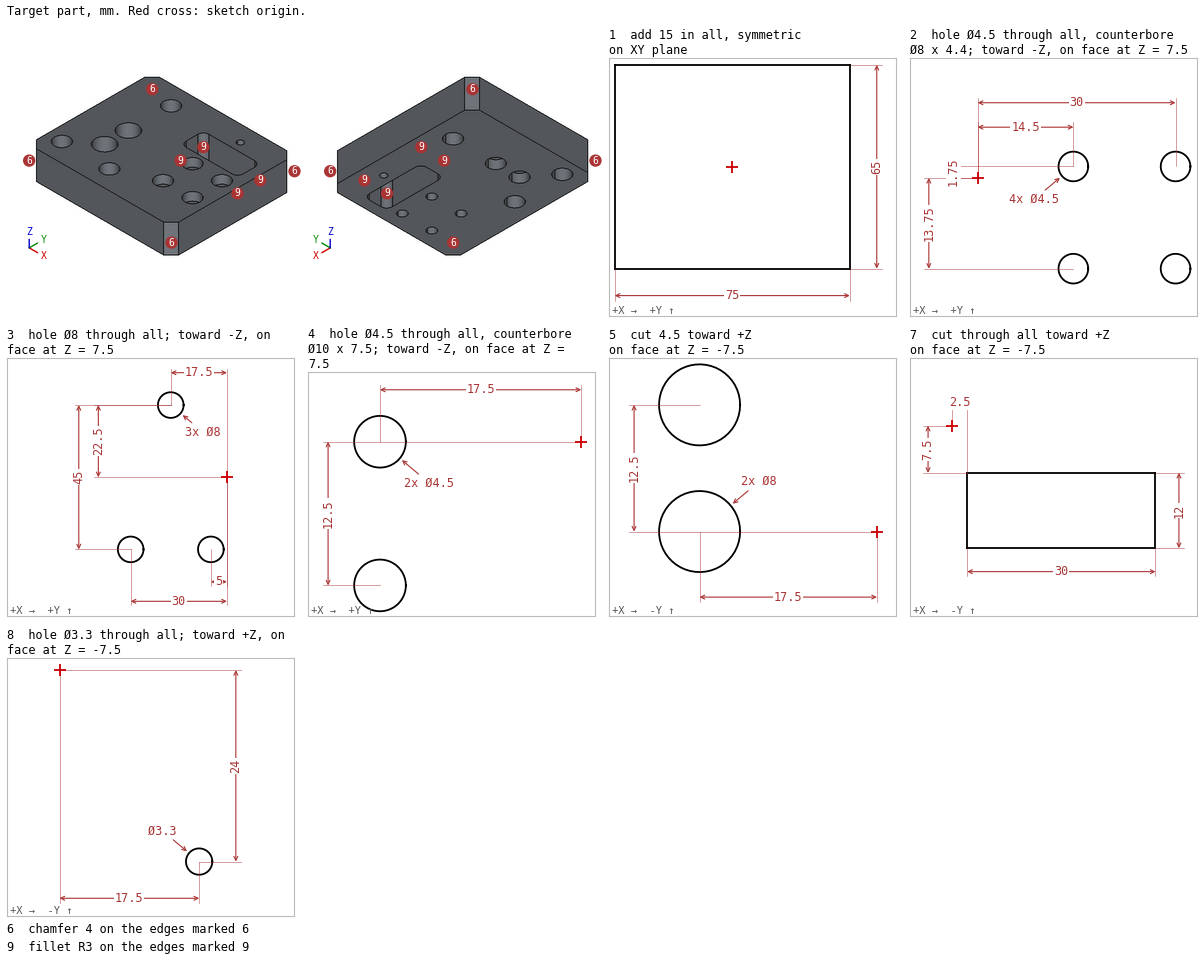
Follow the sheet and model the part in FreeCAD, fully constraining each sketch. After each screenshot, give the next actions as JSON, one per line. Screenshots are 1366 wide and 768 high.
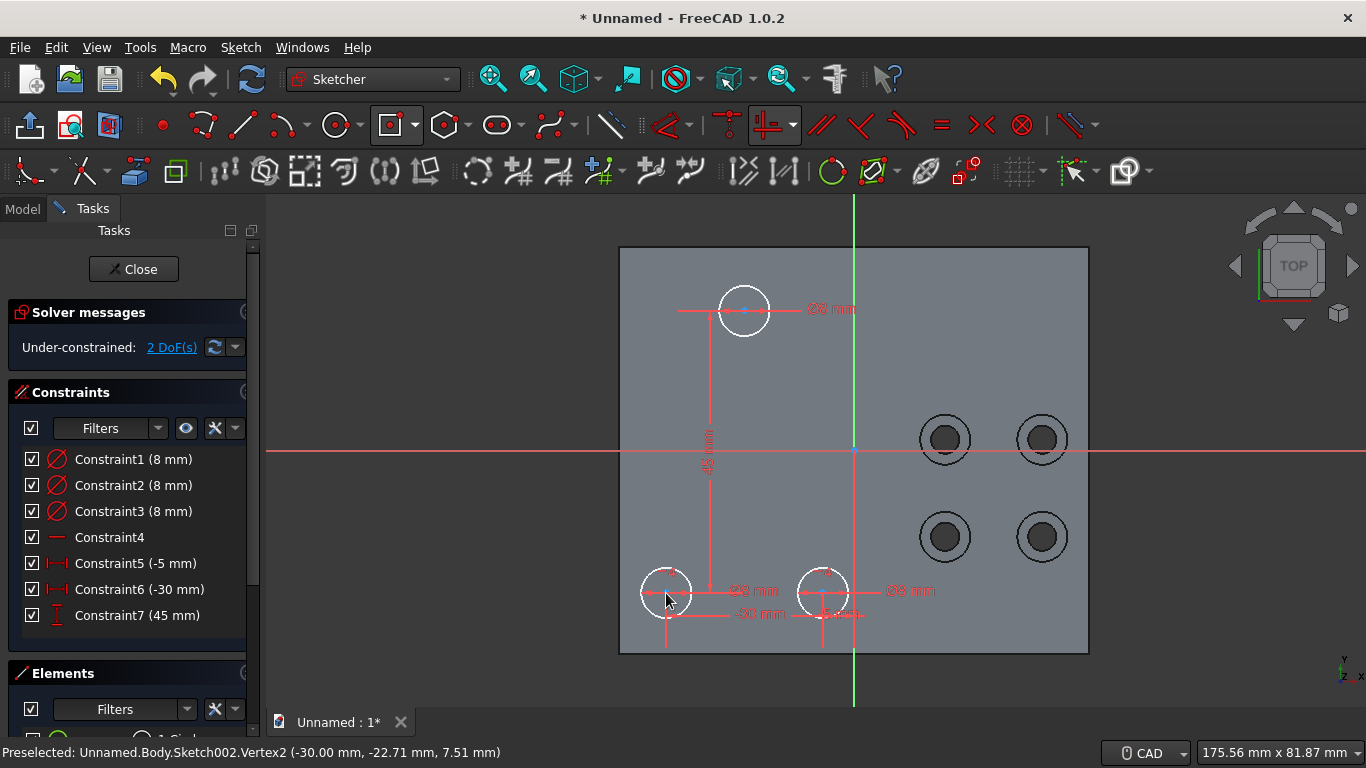
{"action": "left_click", "coordinate": [744, 311]}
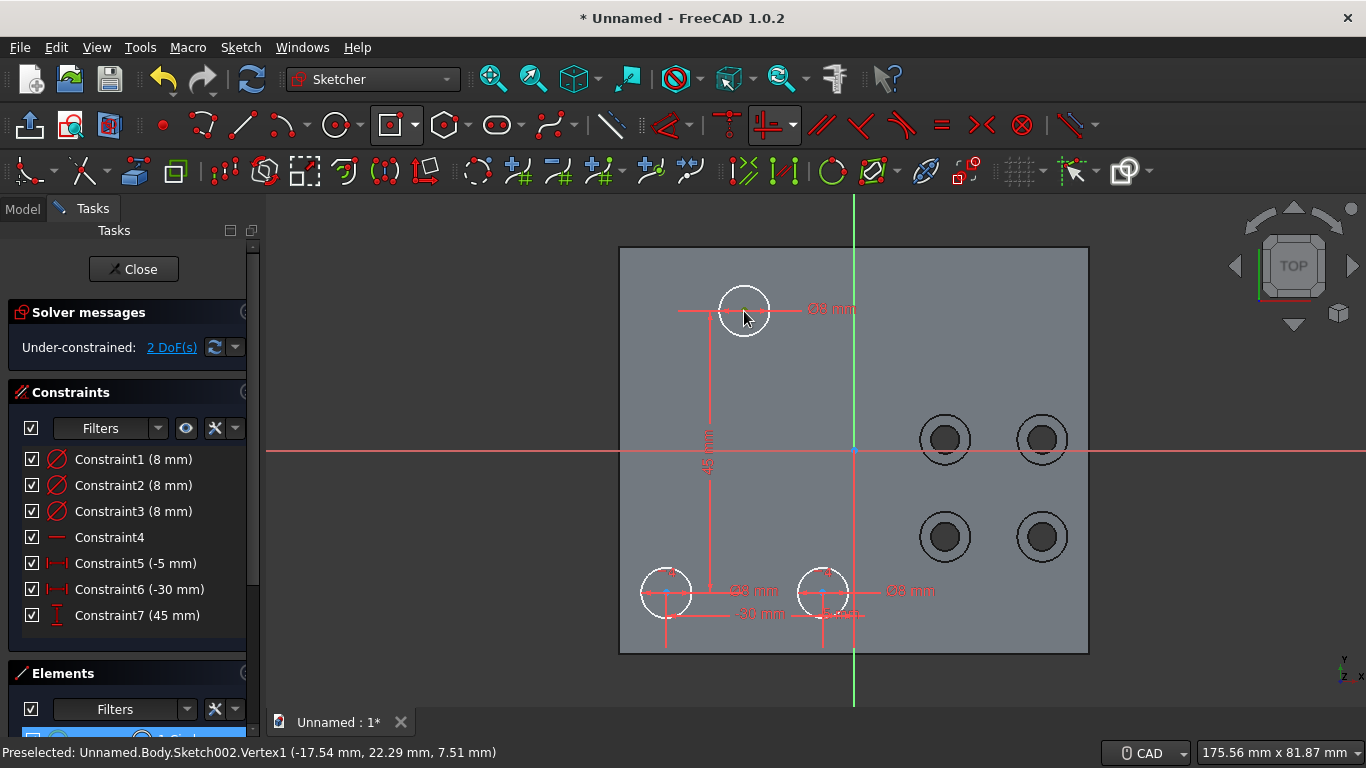
{"action": "key", "text": "l"}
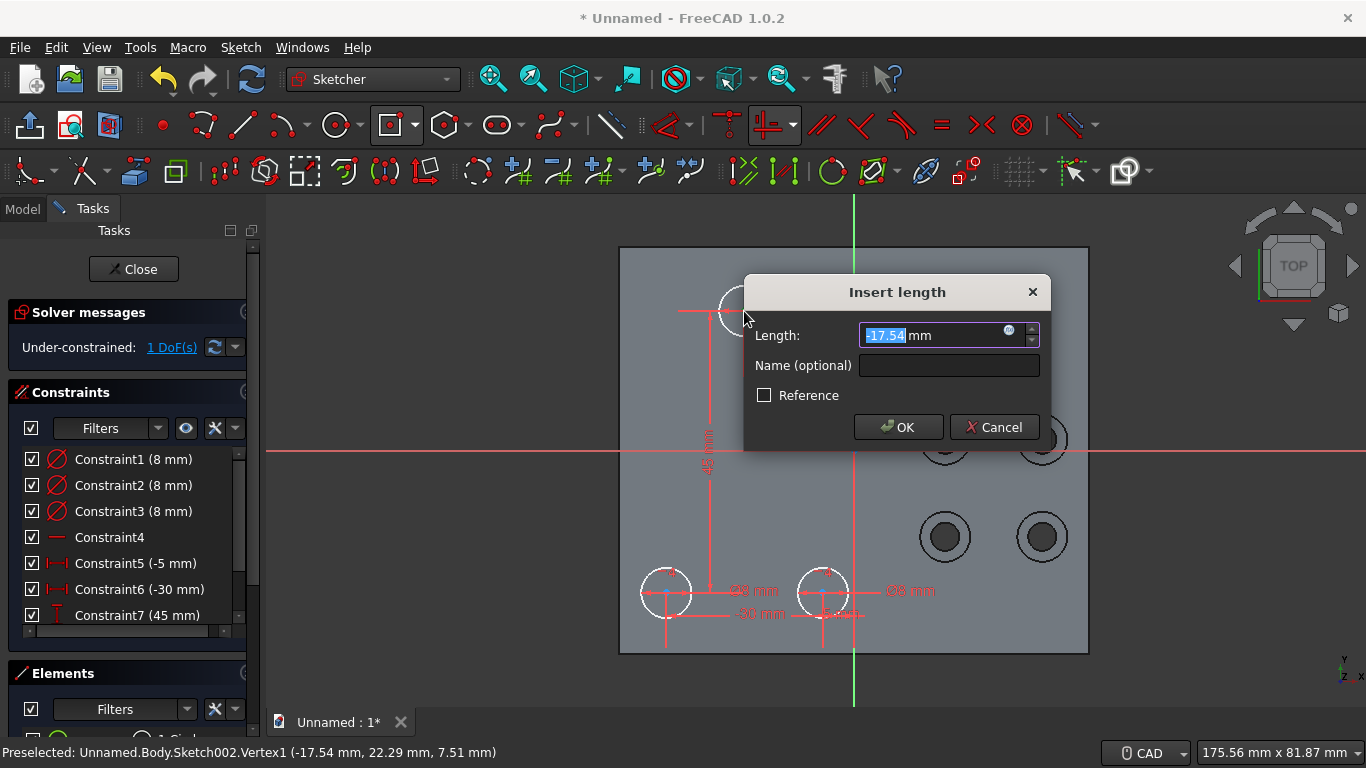
{"action": "type", "text": "-17.5"}
{"action": "key", "text": "Return"}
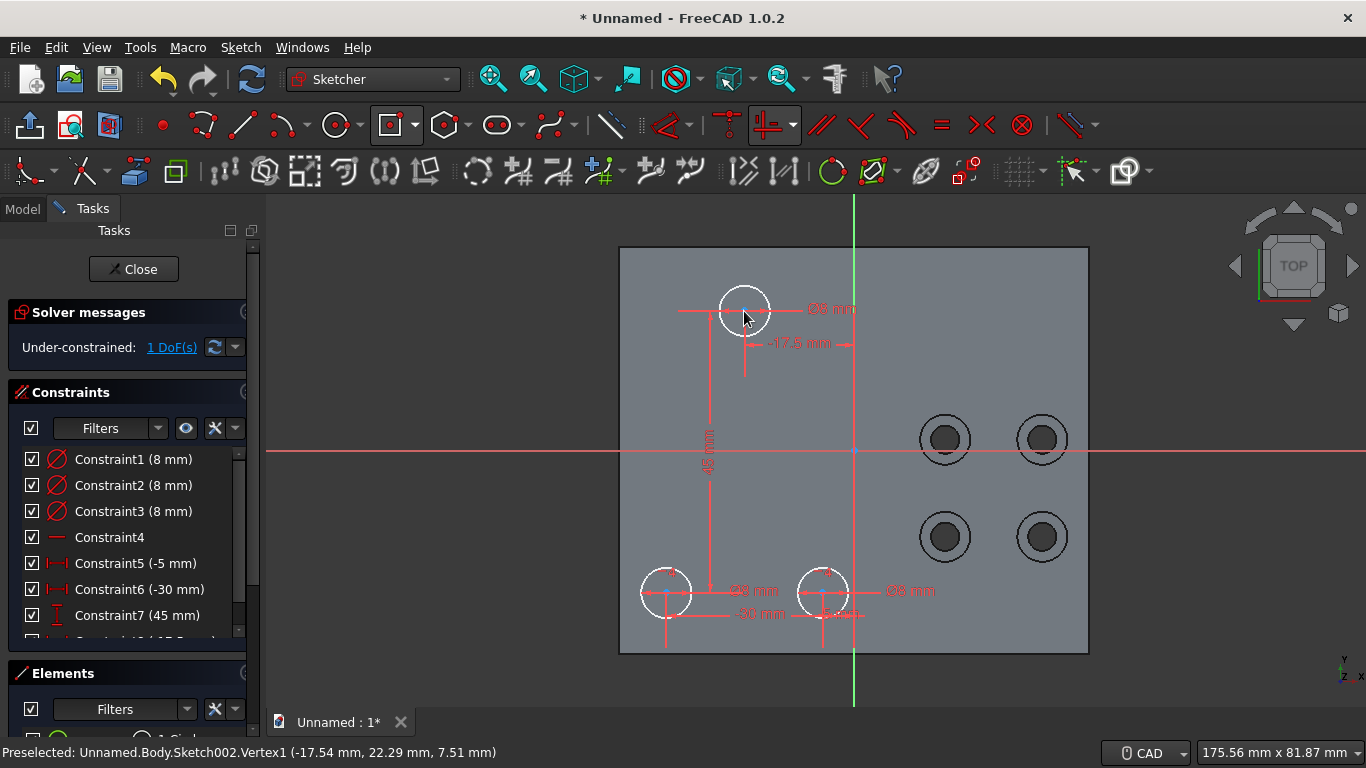
{"action": "left_click", "coordinate": [745, 311]}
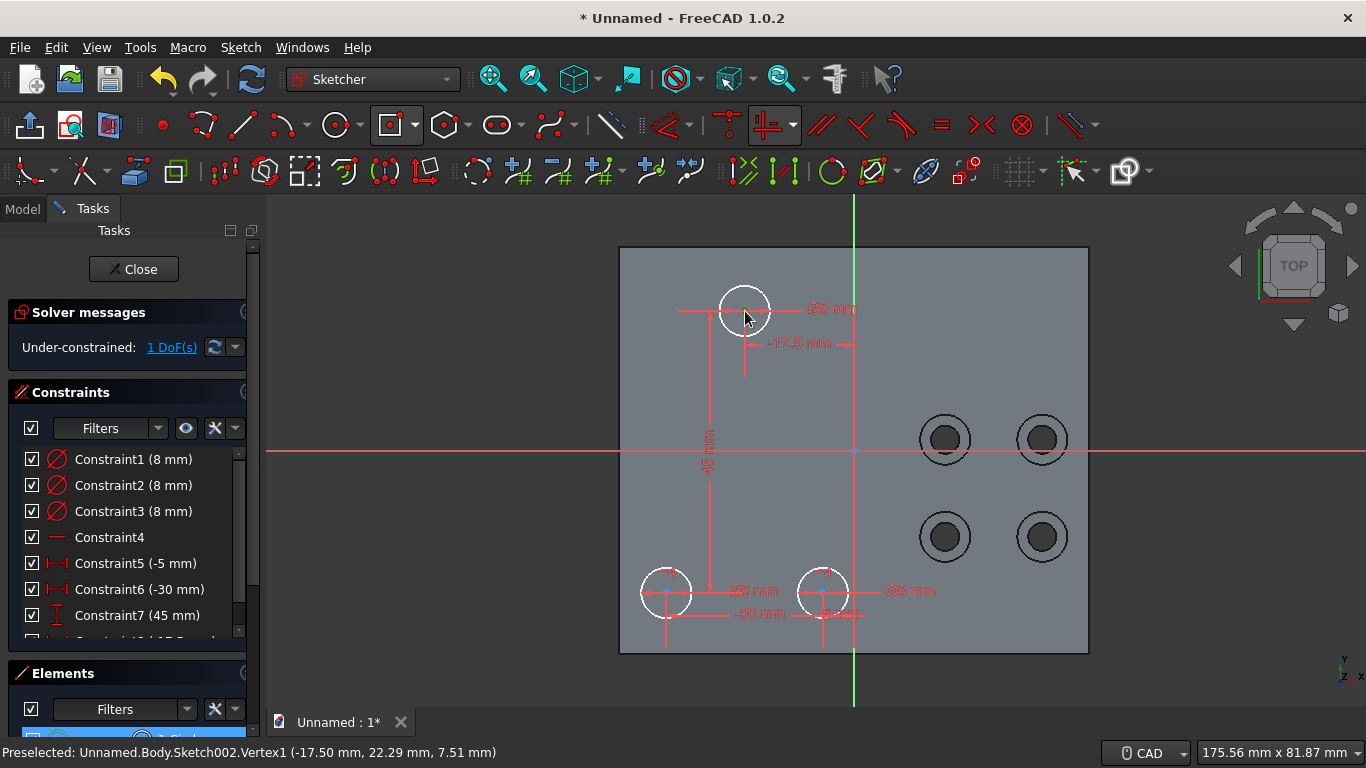
{"action": "key", "text": "i"}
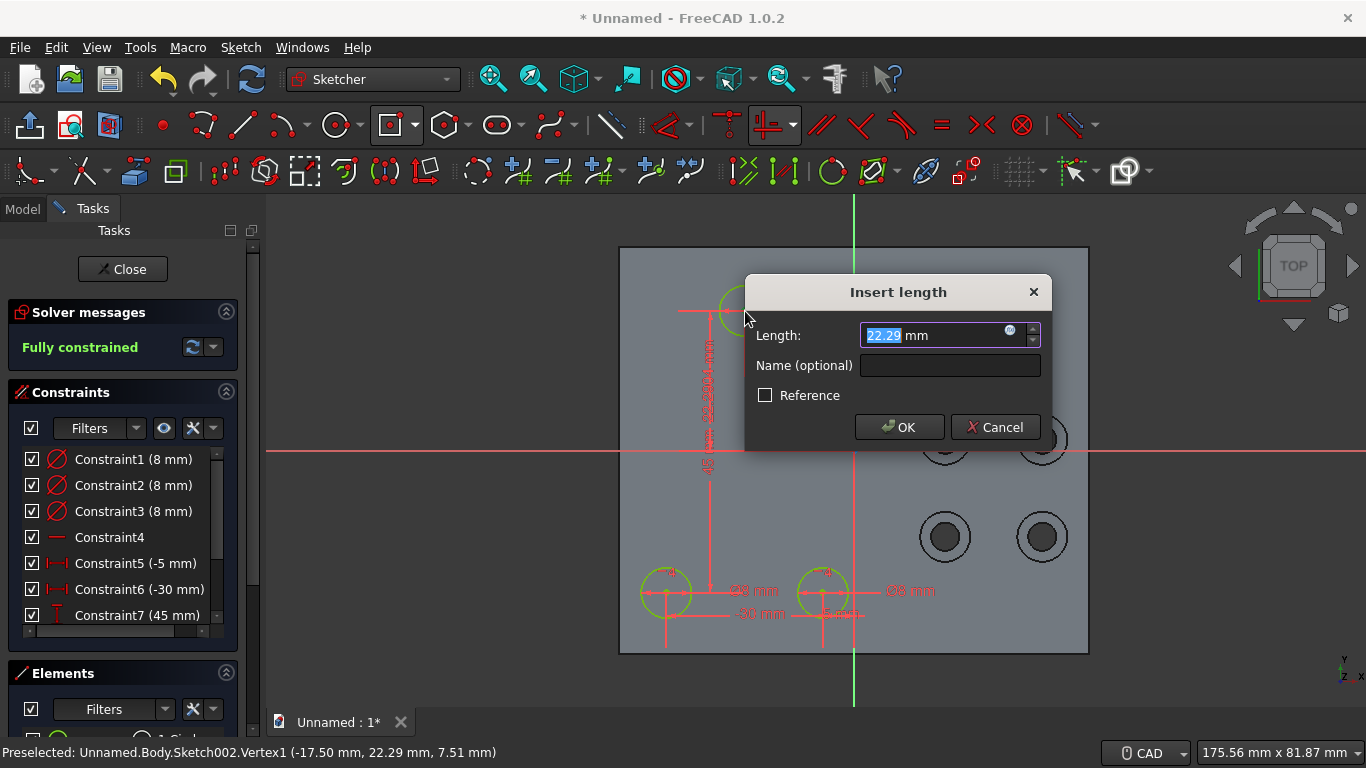
{"action": "type", "text": "22.5"}
{"action": "key", "text": "Return"}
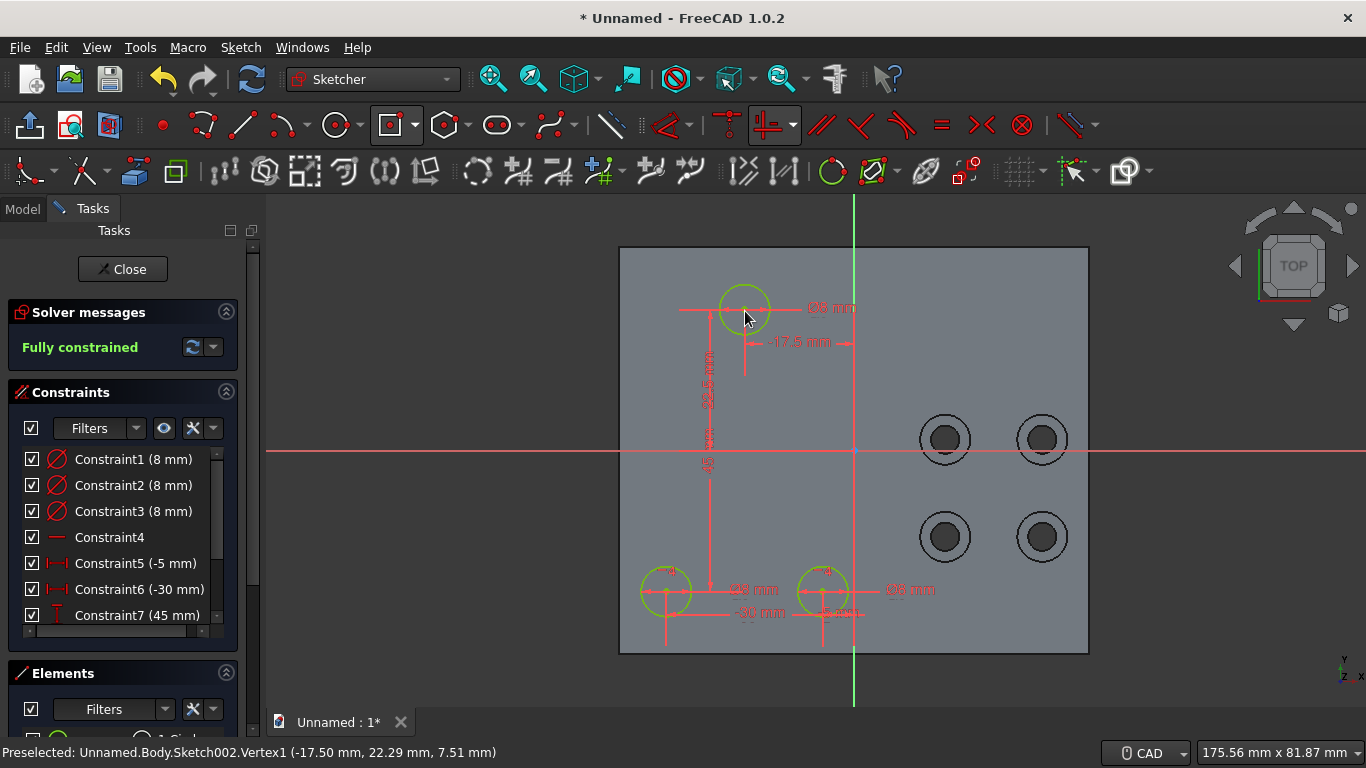
{"action": "left_click", "coordinate": [123, 269]}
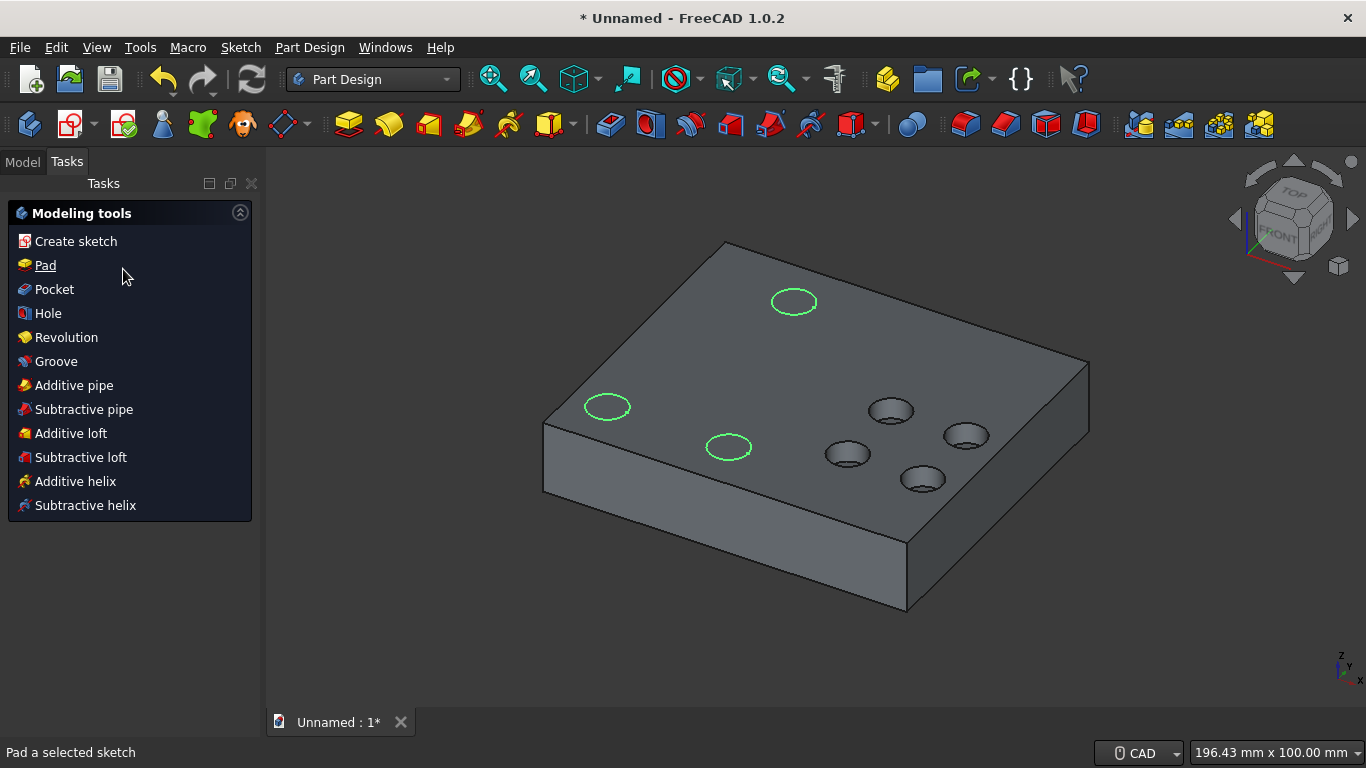
{"action": "left_click", "coordinate": [652, 124]}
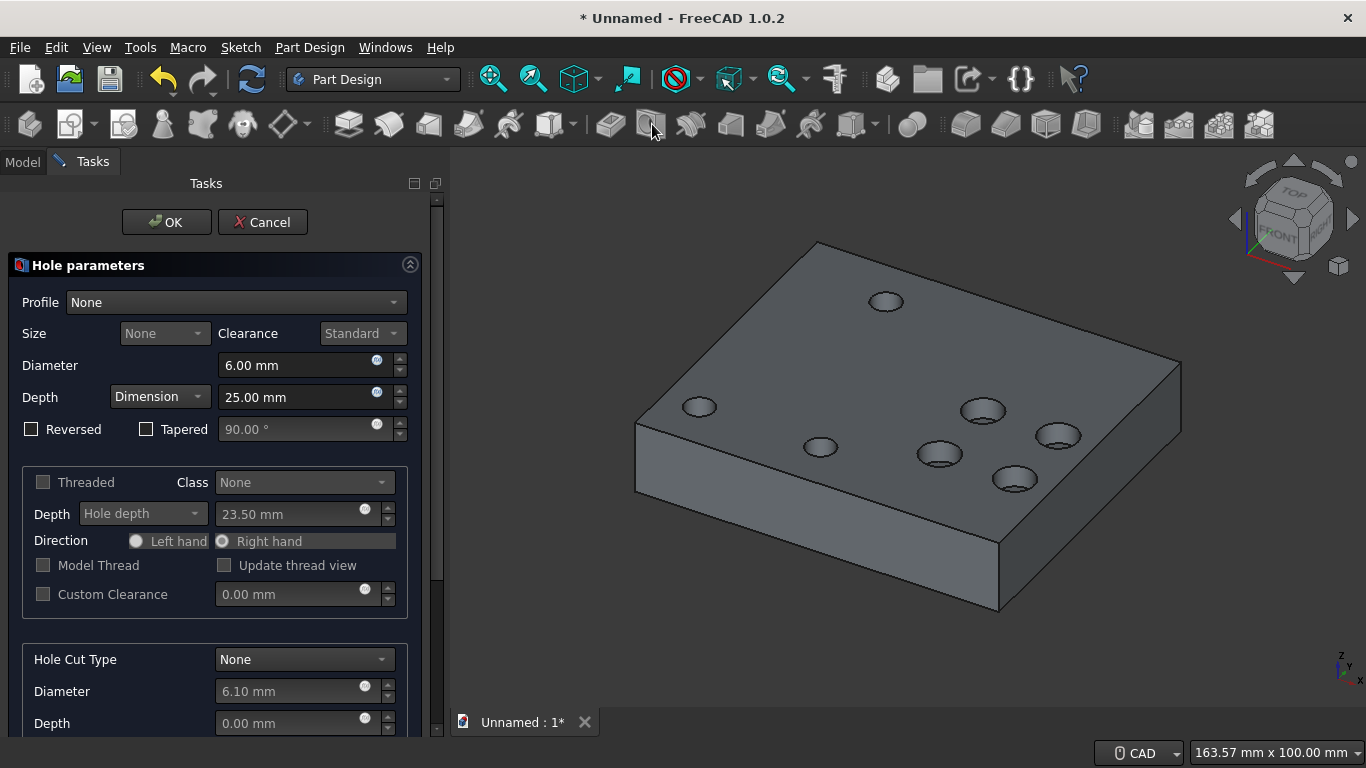
{"action": "triple_click", "coordinate": [305, 365]}